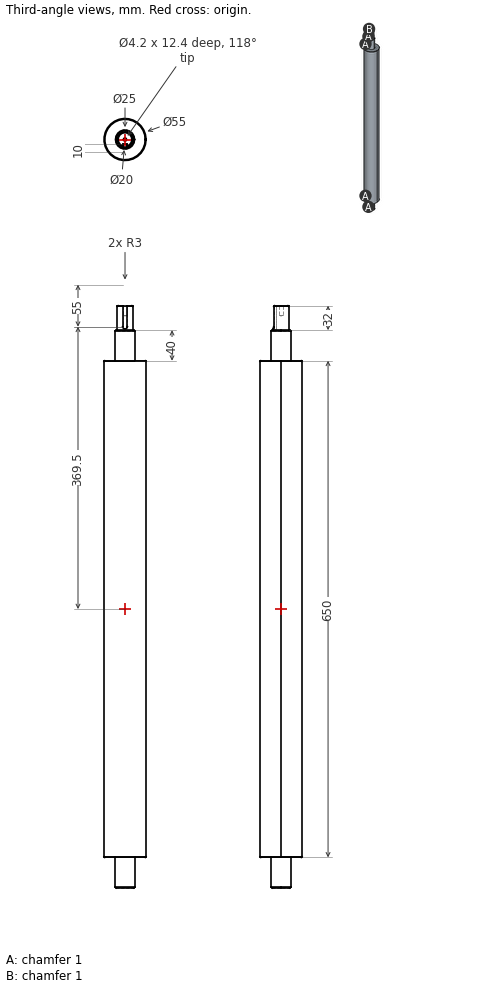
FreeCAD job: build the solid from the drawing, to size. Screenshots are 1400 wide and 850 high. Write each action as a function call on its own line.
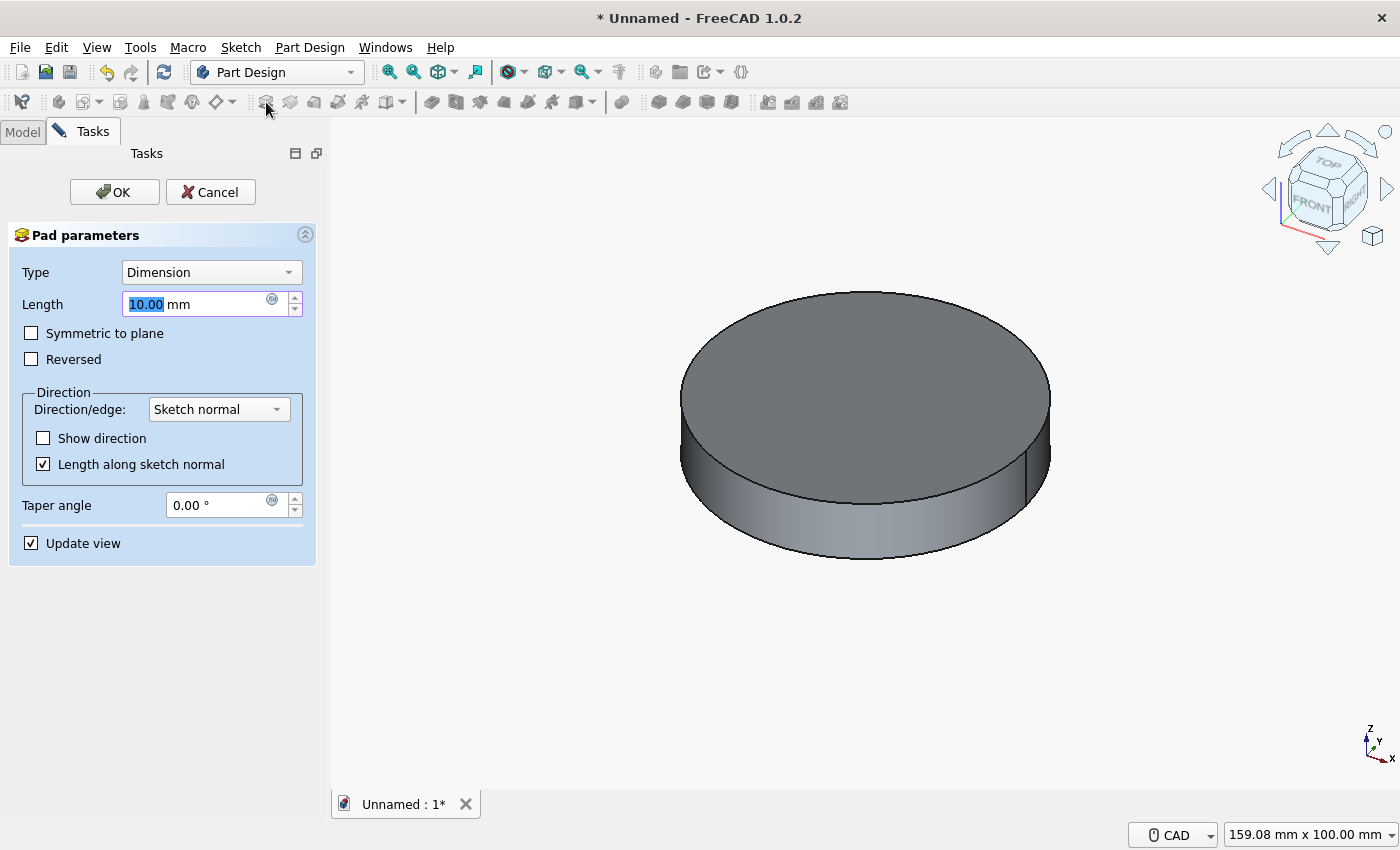
text(650)
key(Tab)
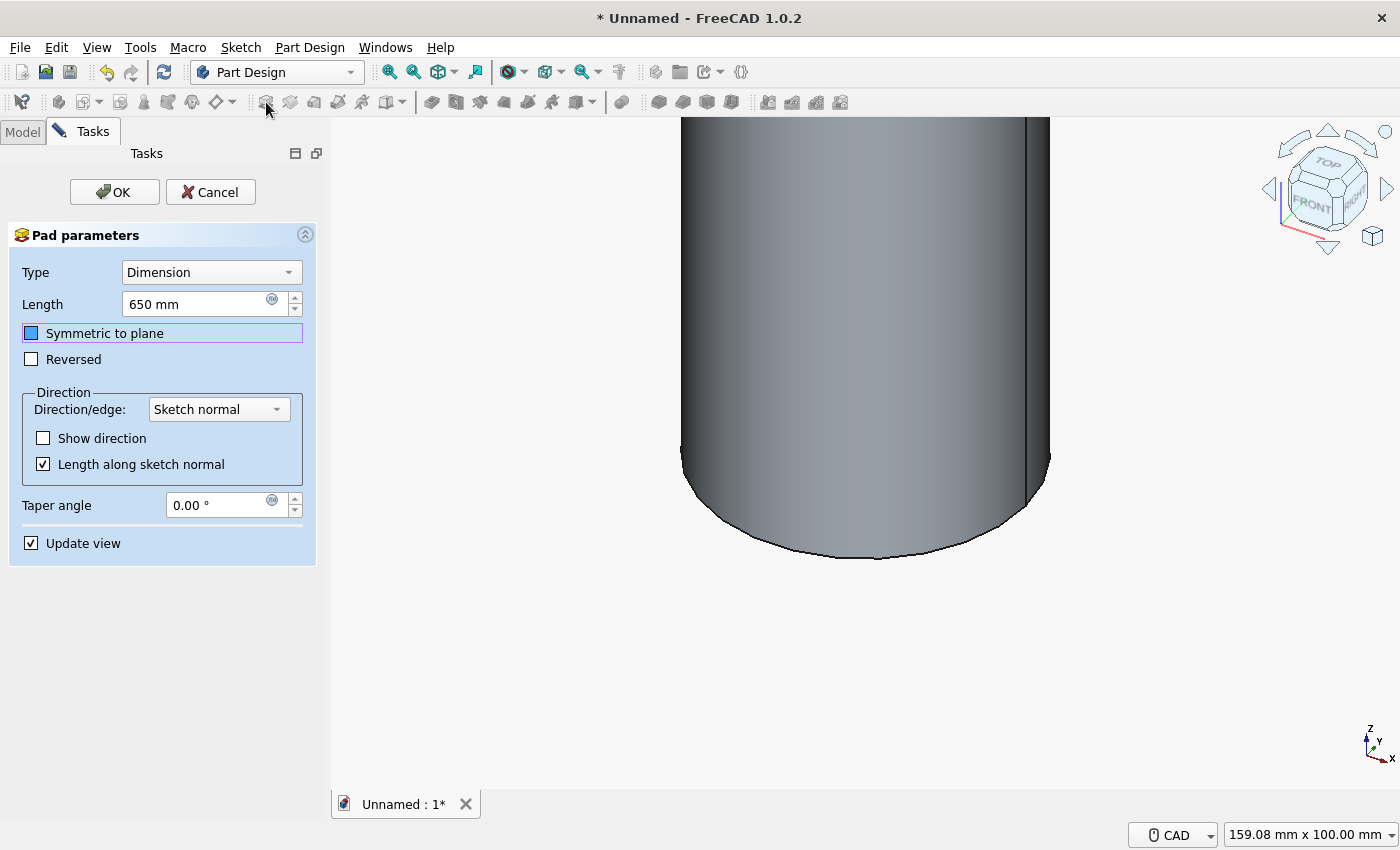
click(30, 333)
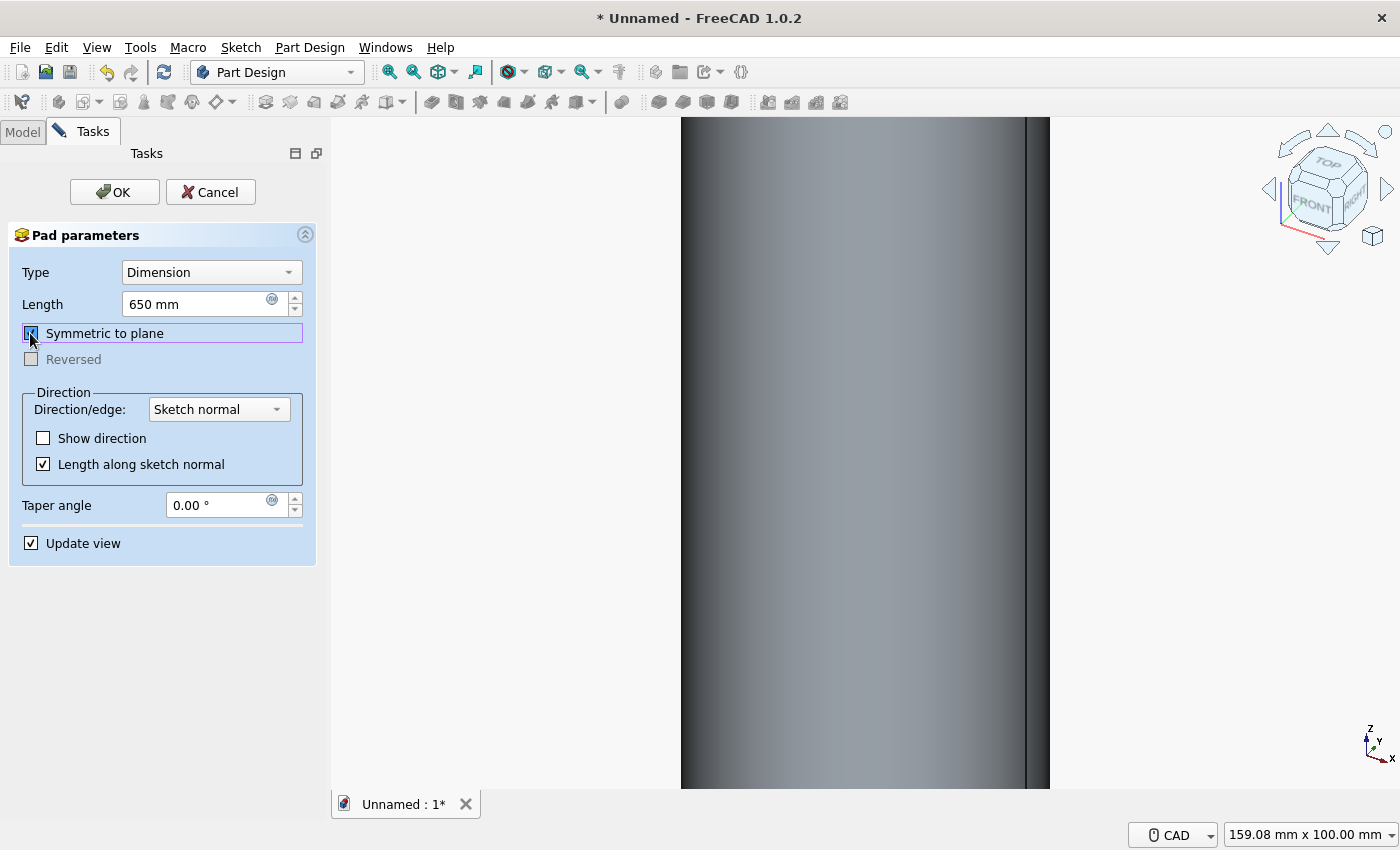
click(115, 192)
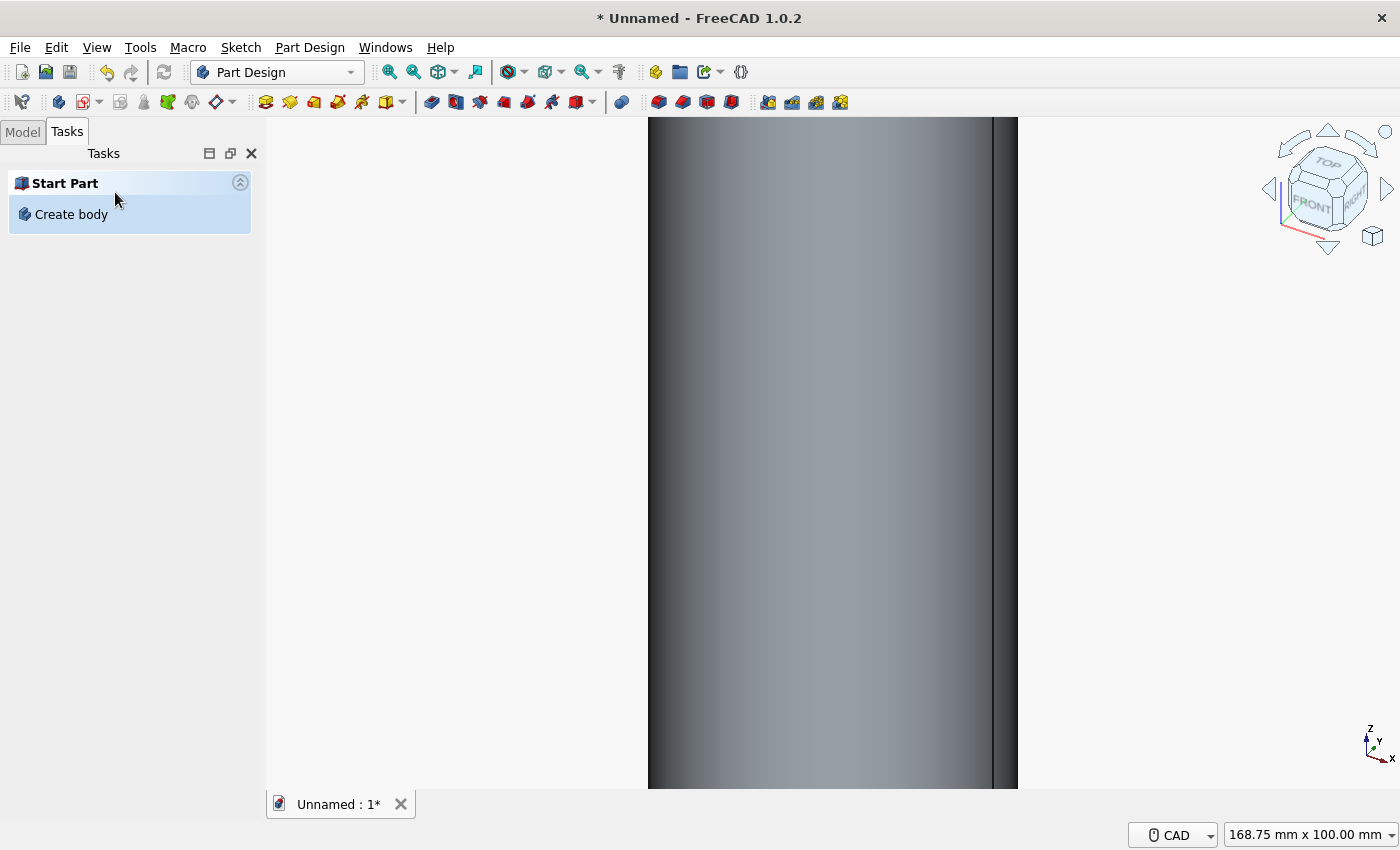
click(390, 72)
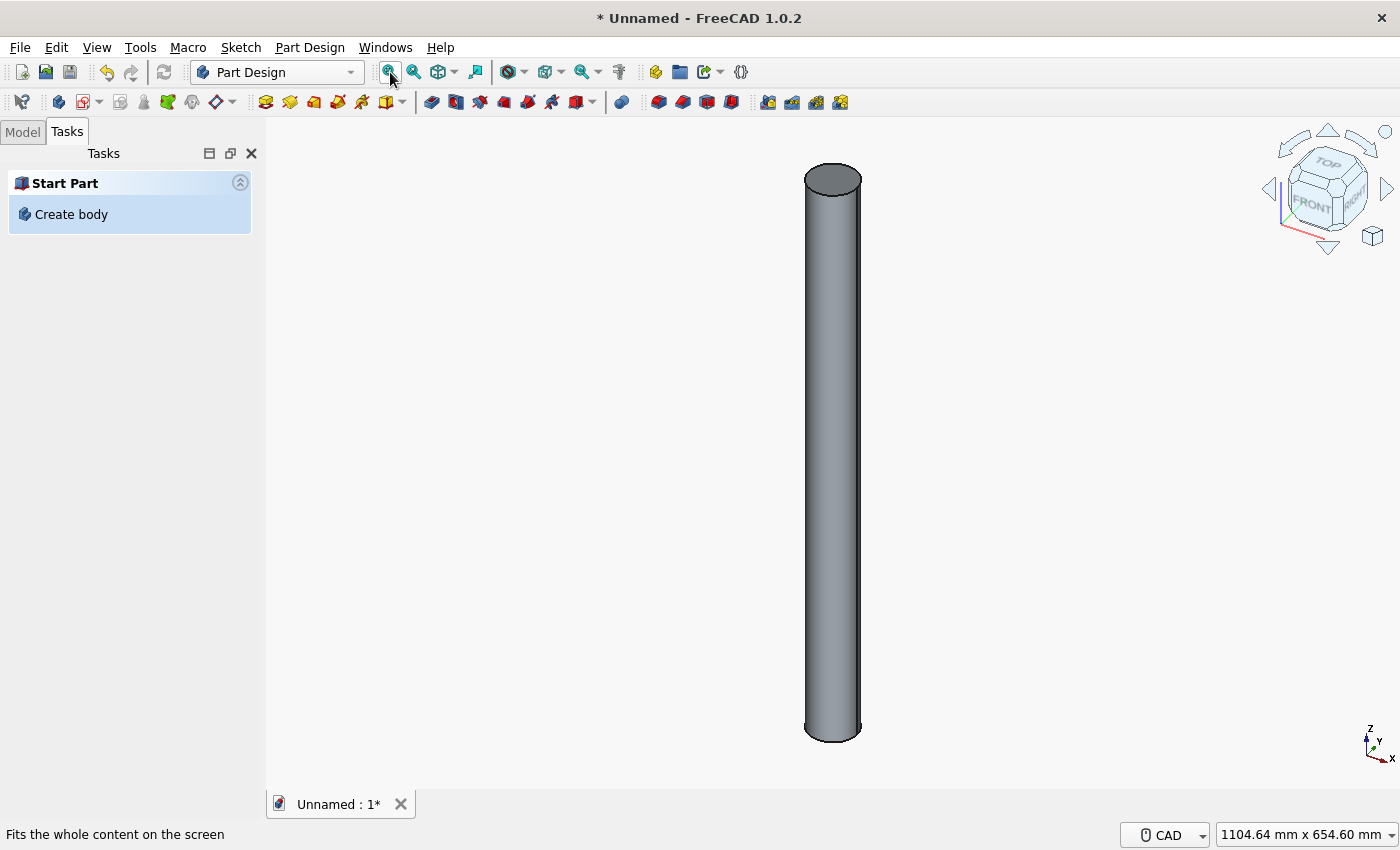
click(833, 179)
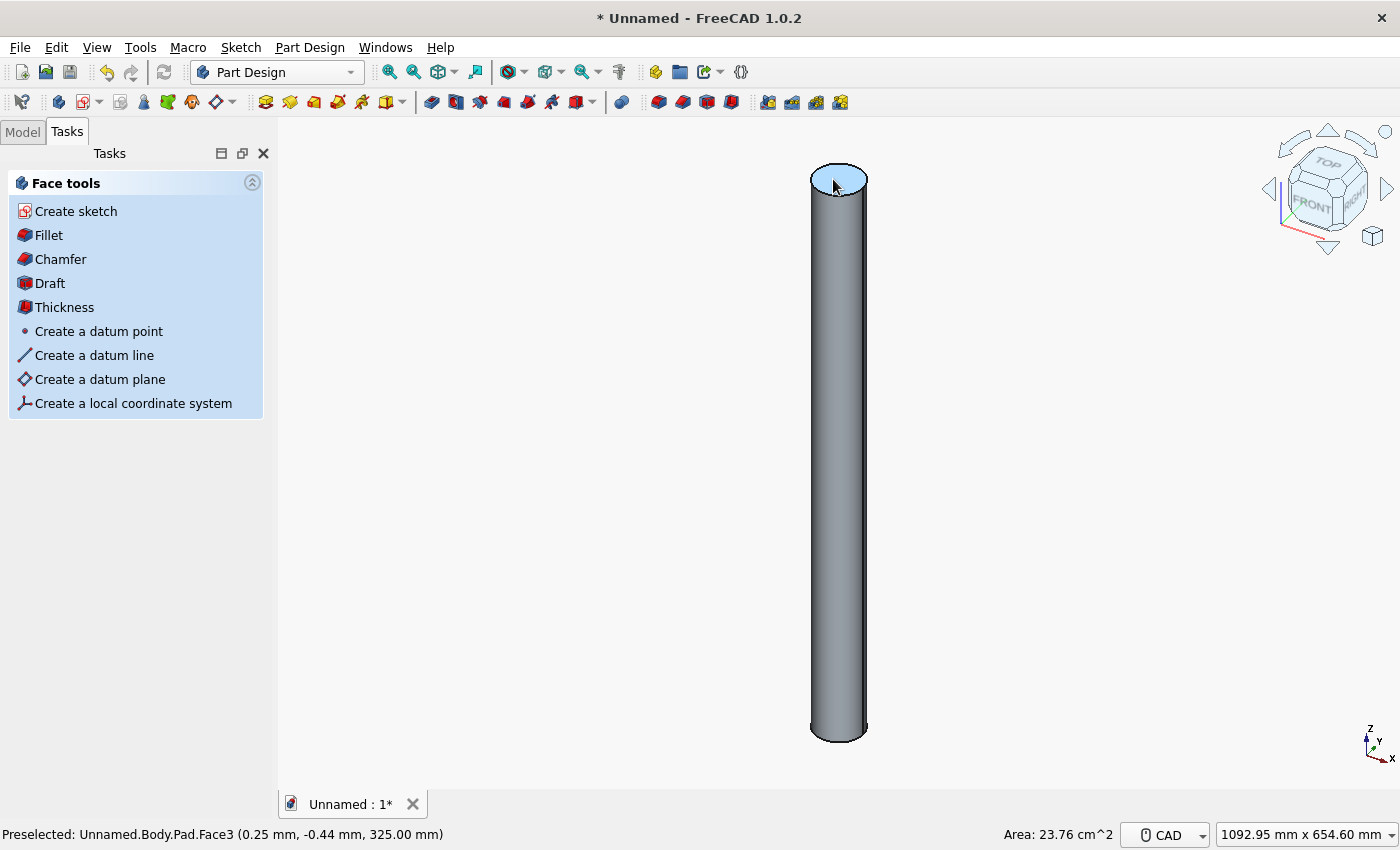
click(84, 102)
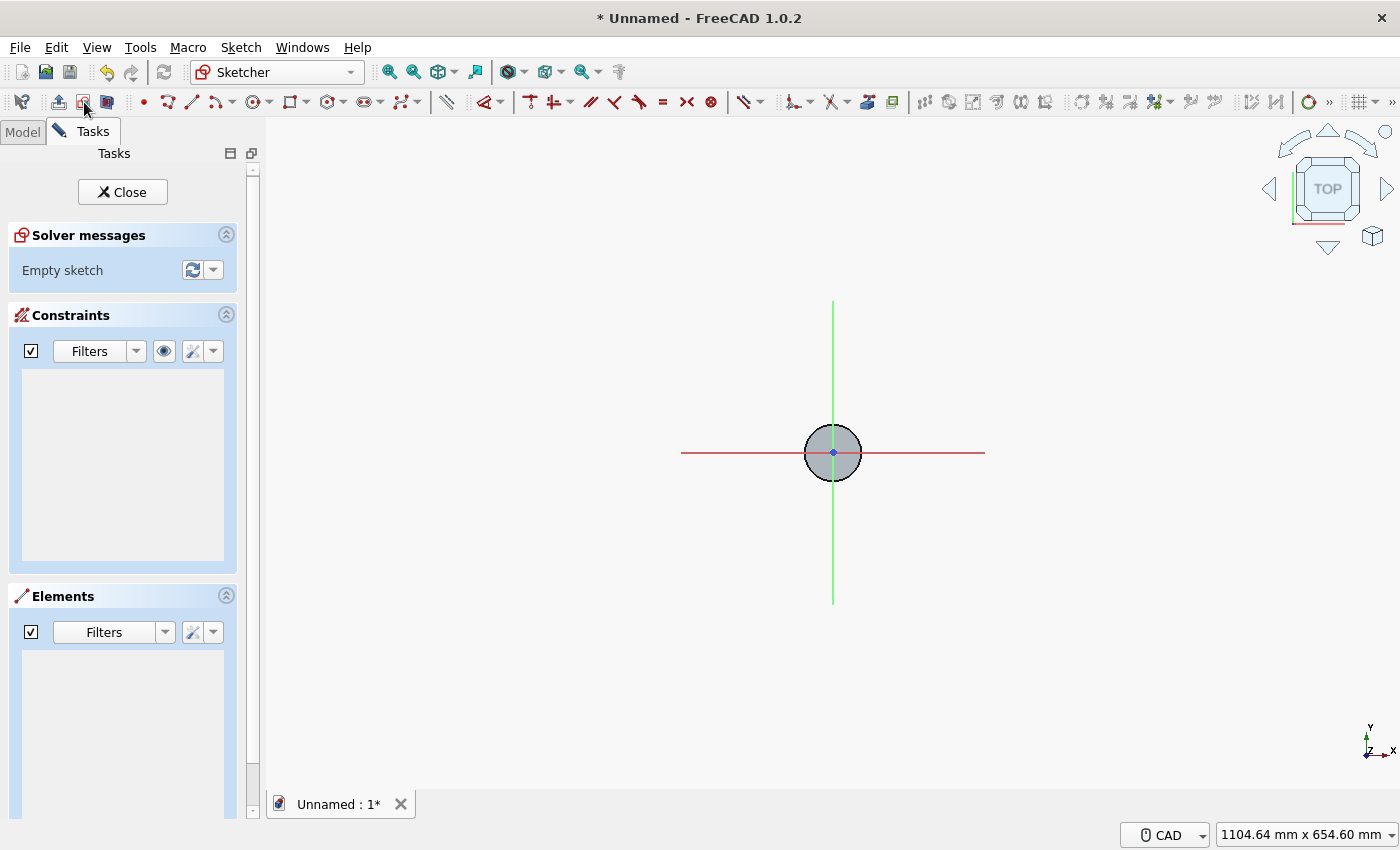
scroll(837, 453, up, 14)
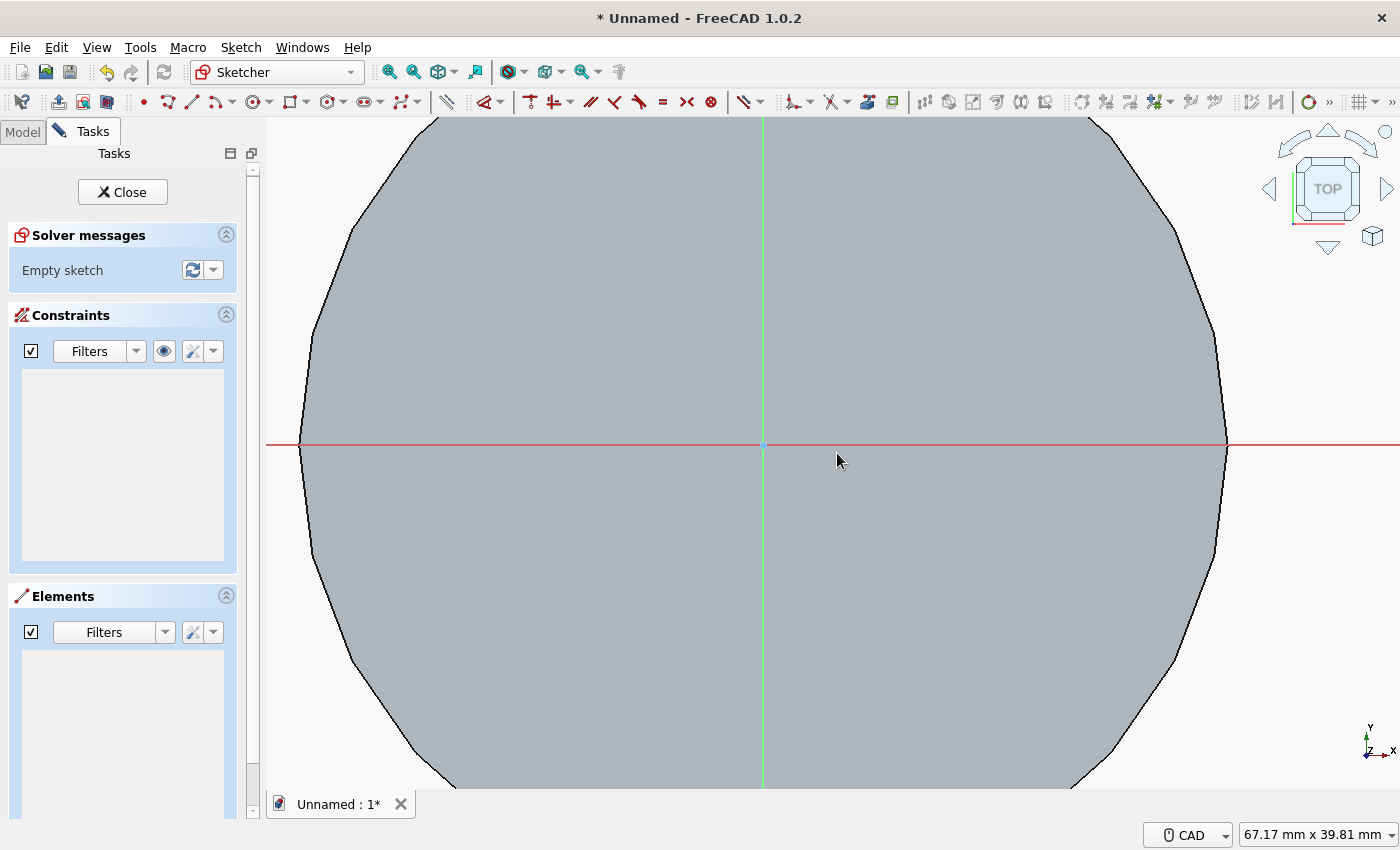
click(254, 102)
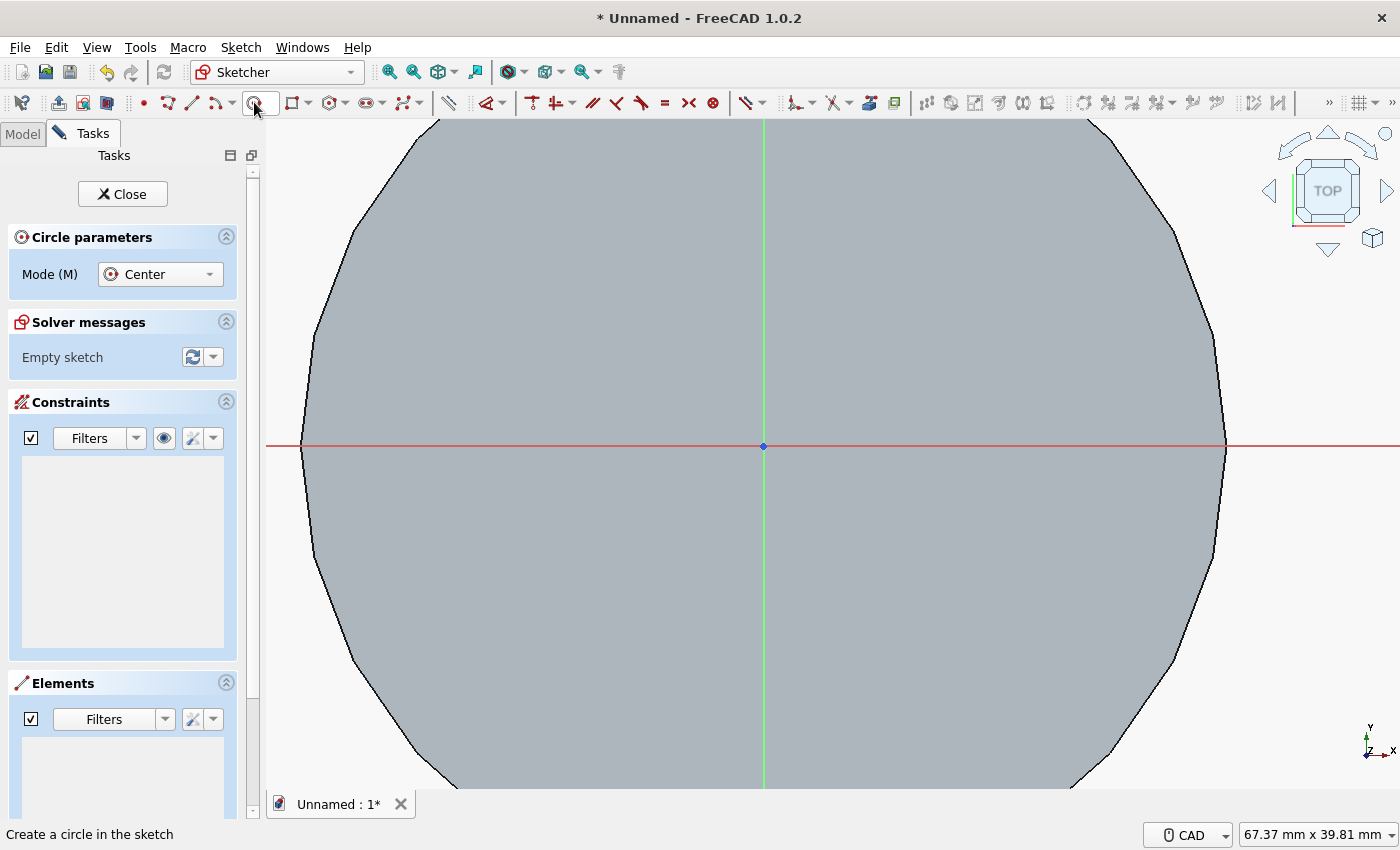
click(764, 446)
move(912, 298)